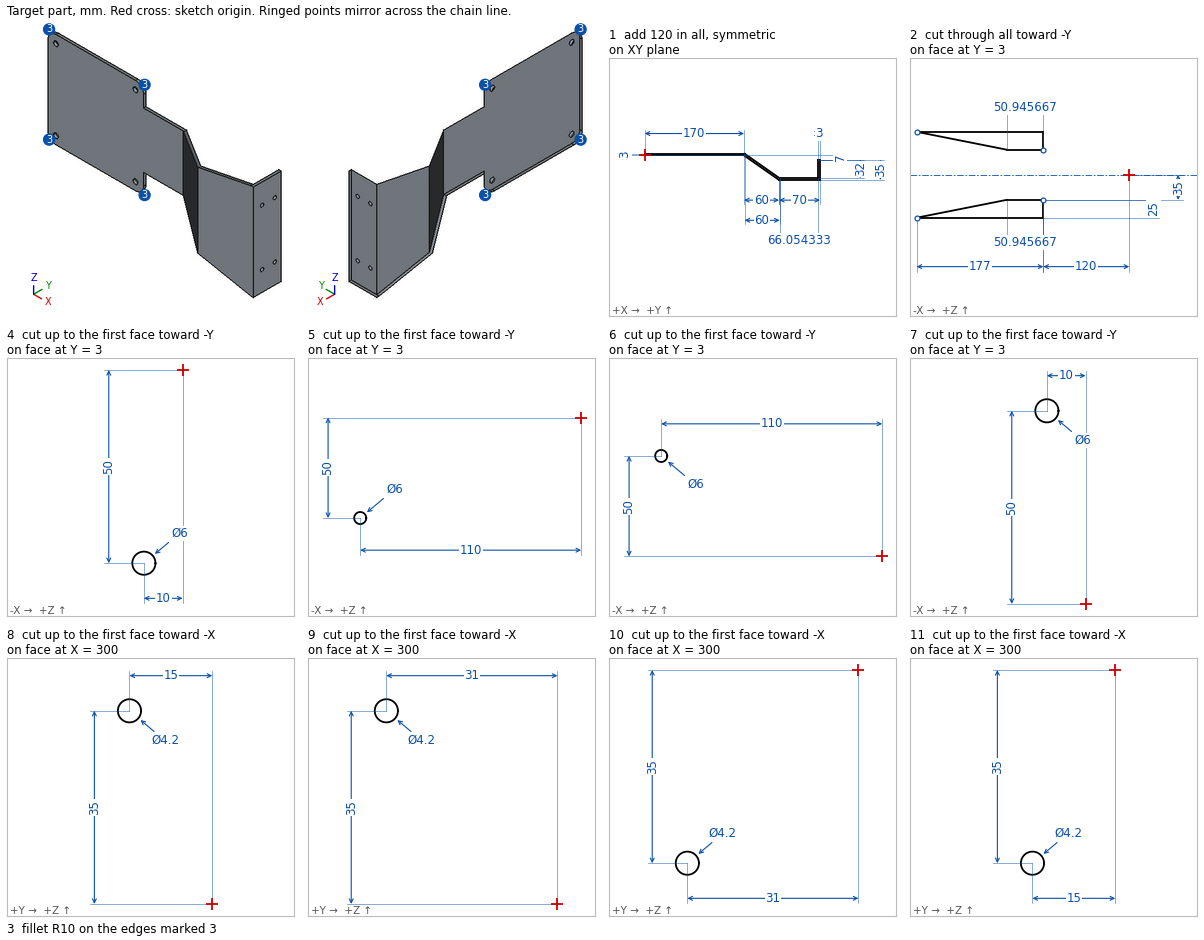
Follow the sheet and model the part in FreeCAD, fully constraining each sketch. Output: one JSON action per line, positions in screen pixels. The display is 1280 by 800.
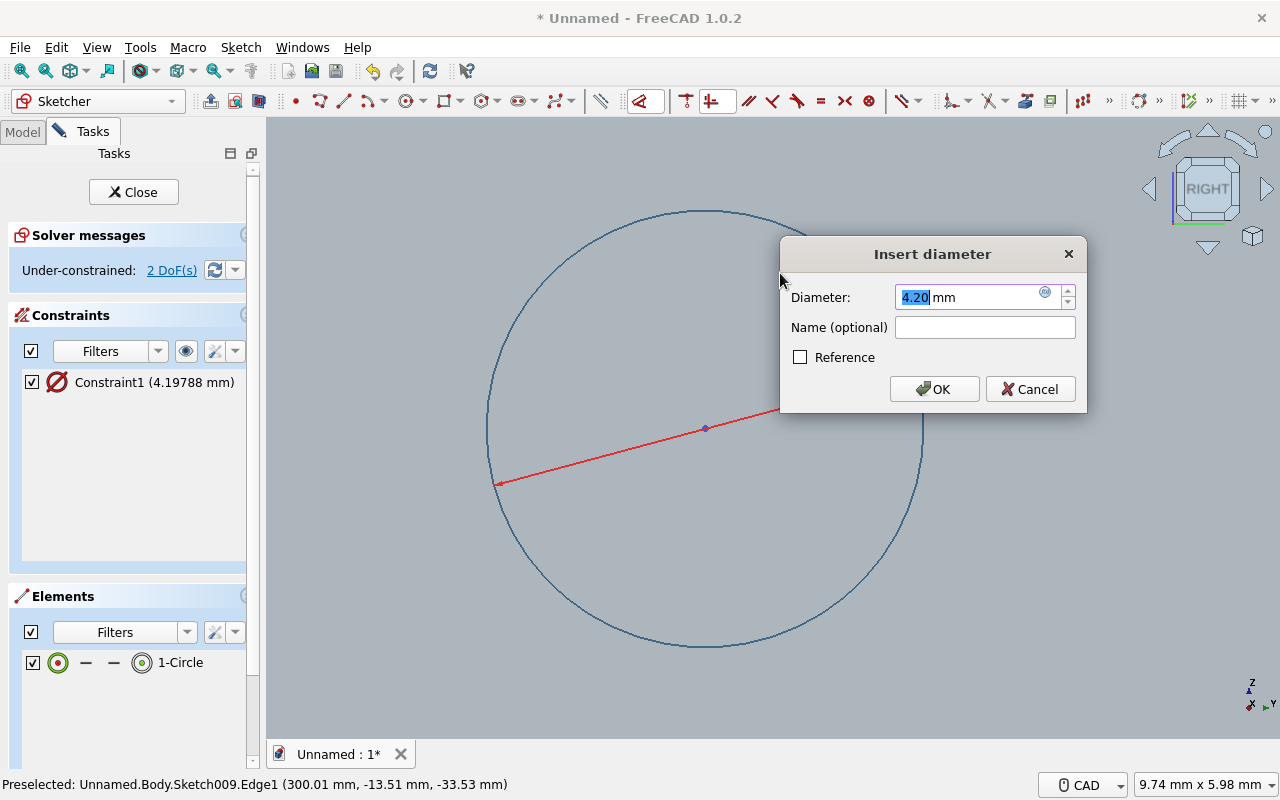
{"action": "type", "text": "4.2"}
{"action": "key", "text": "Return"}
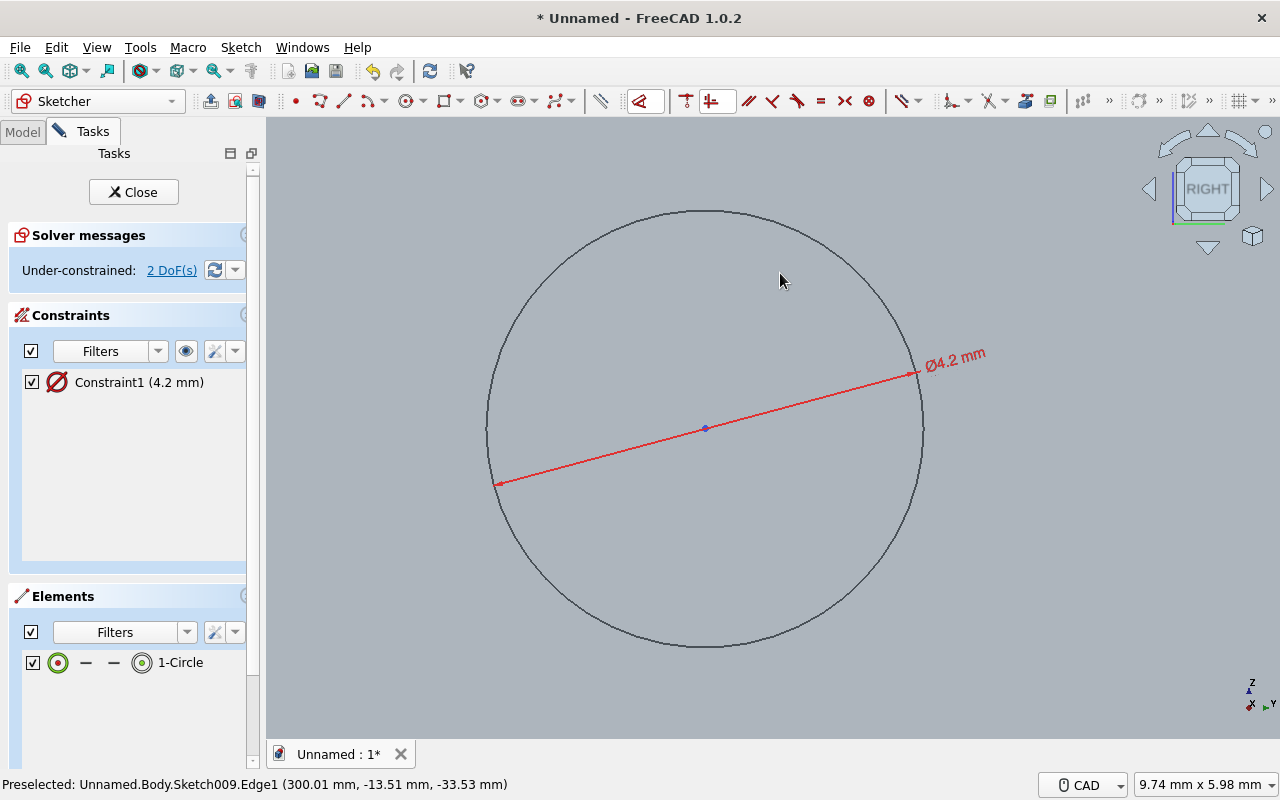
{"action": "left_click", "coordinate": [705, 429]}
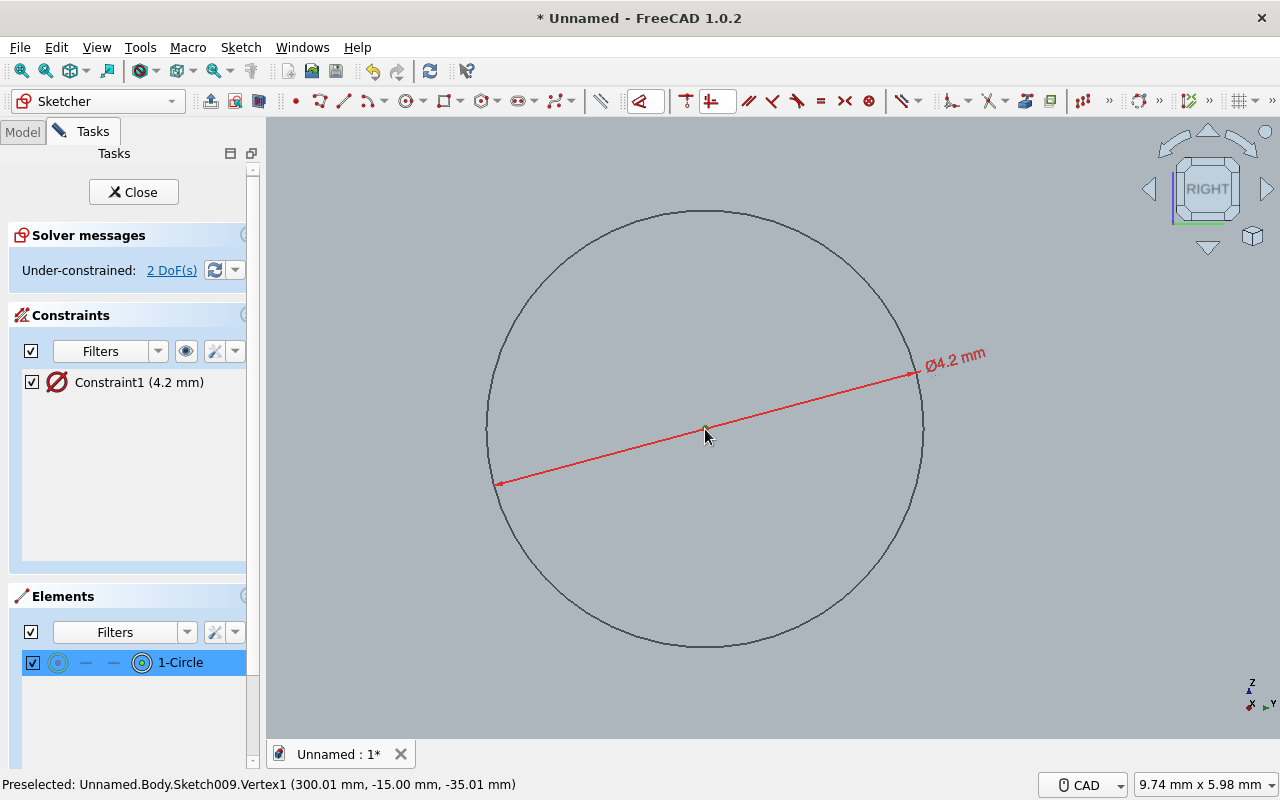
{"action": "key", "text": "l"}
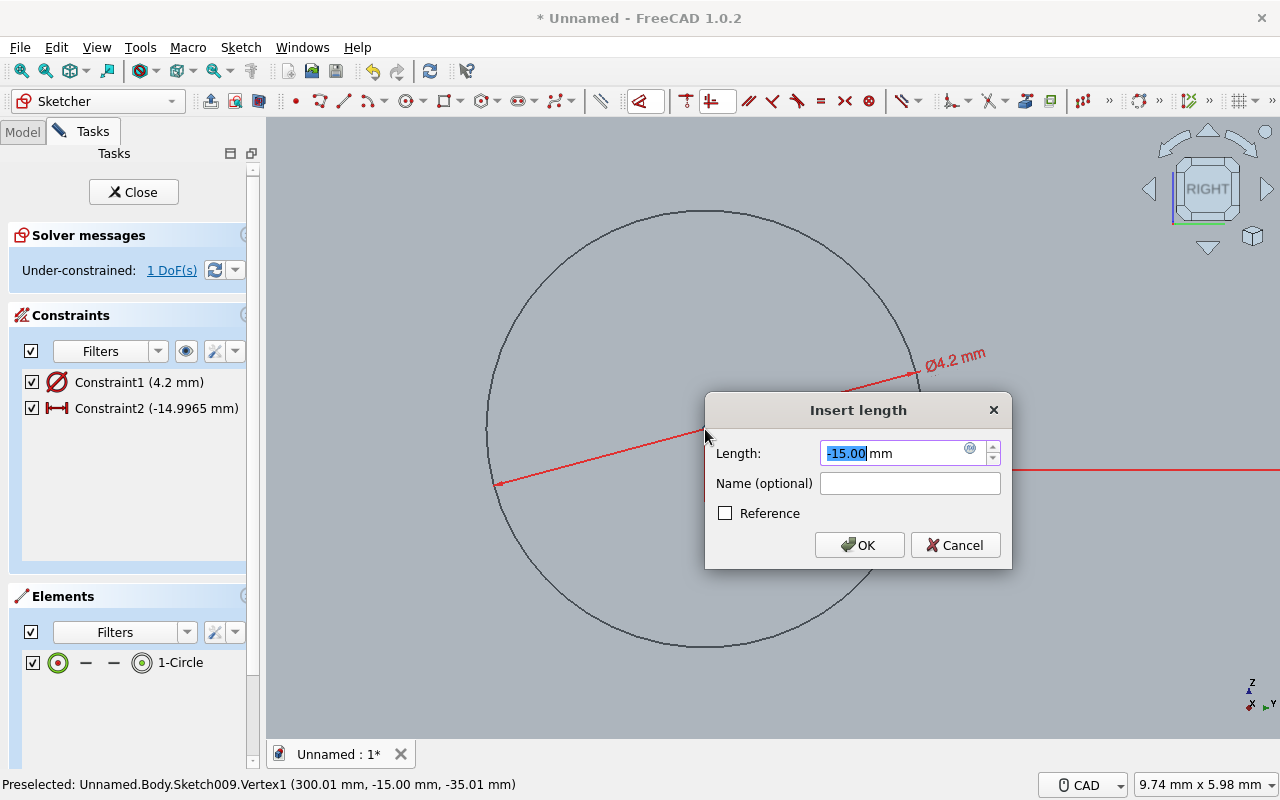
{"action": "type", "text": "-15"}
{"action": "key", "text": "Return"}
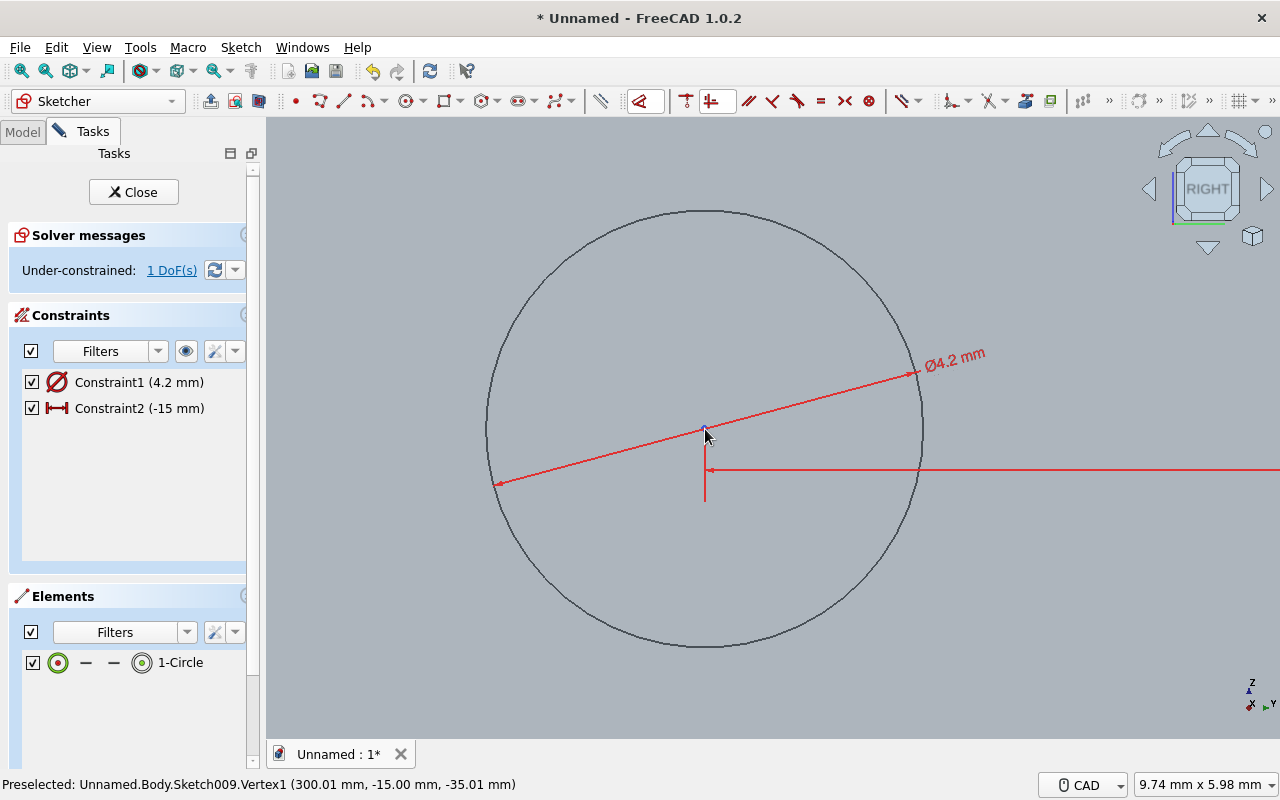
{"action": "left_click", "coordinate": [705, 429]}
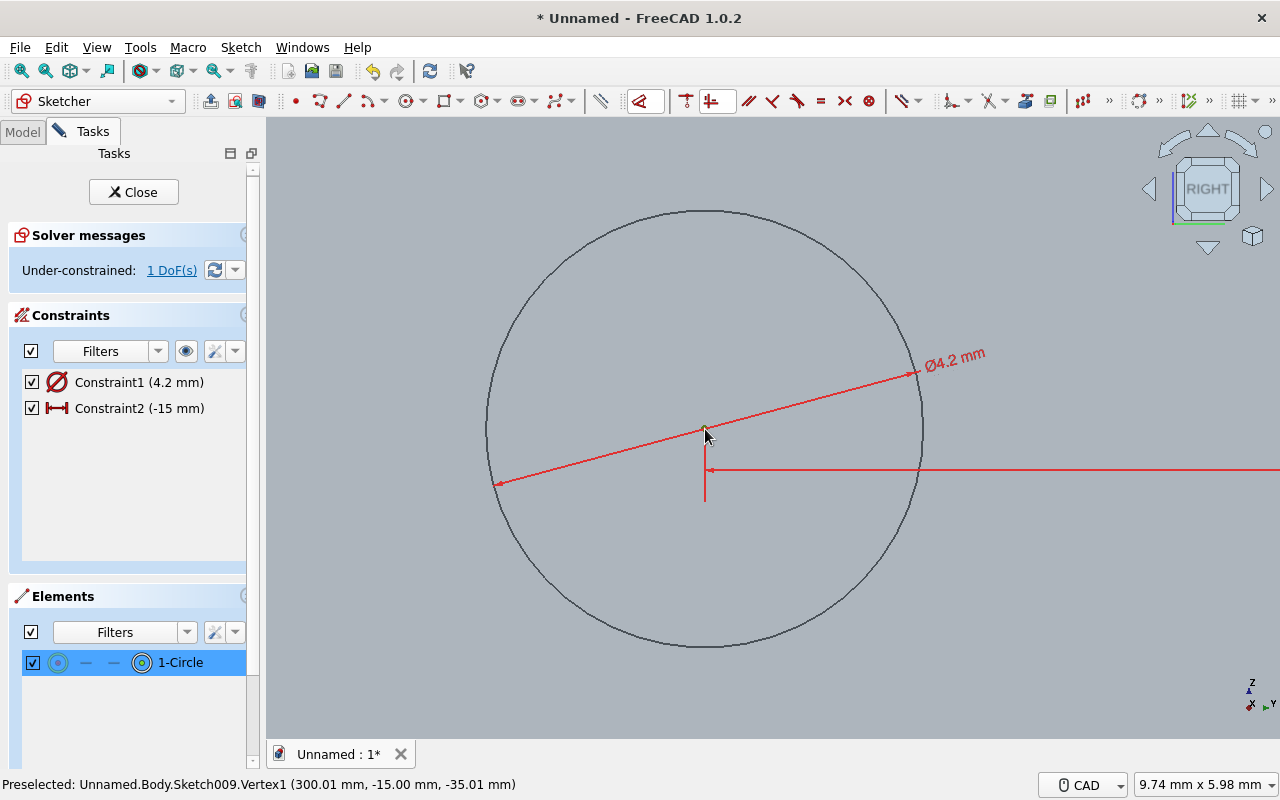
{"action": "left_click", "coordinate": [658, 102]}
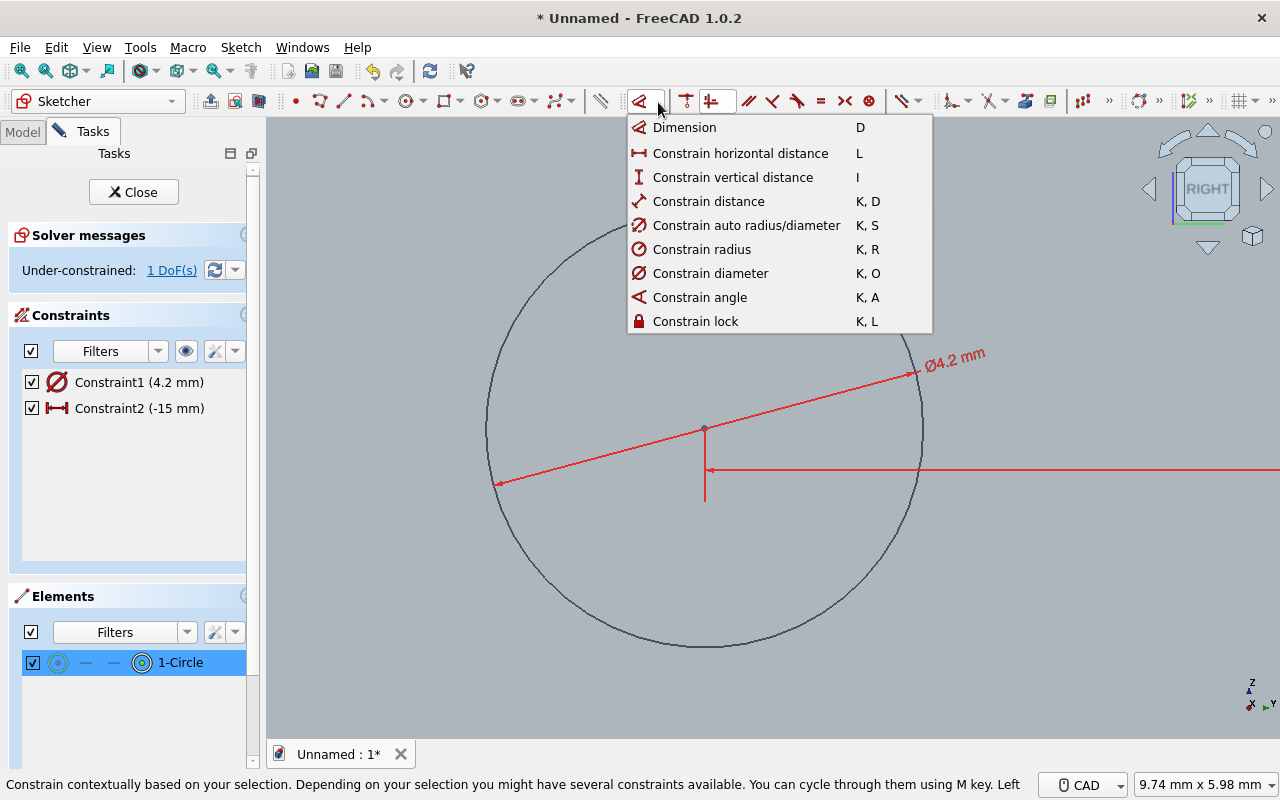
{"action": "left_click", "coordinate": [780, 177]}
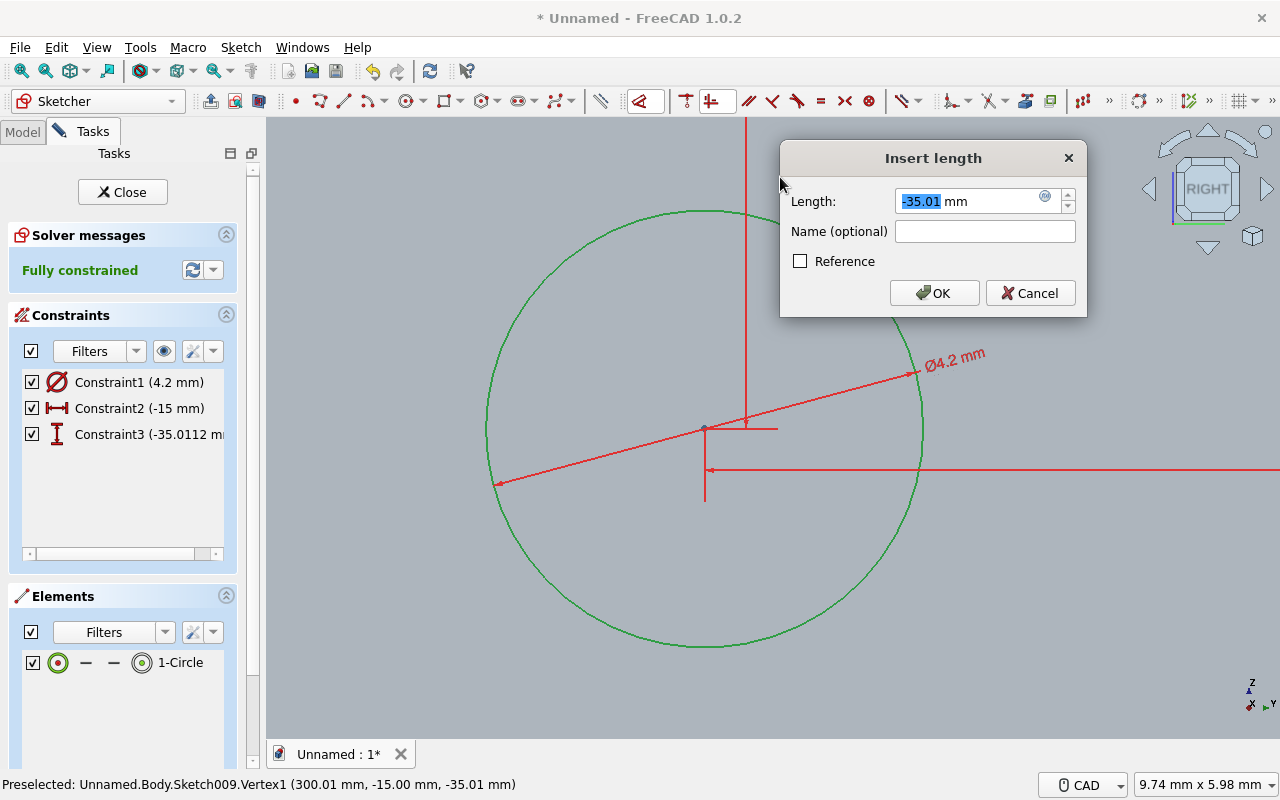
{"action": "type", "text": "-35"}
{"action": "key", "text": "Return"}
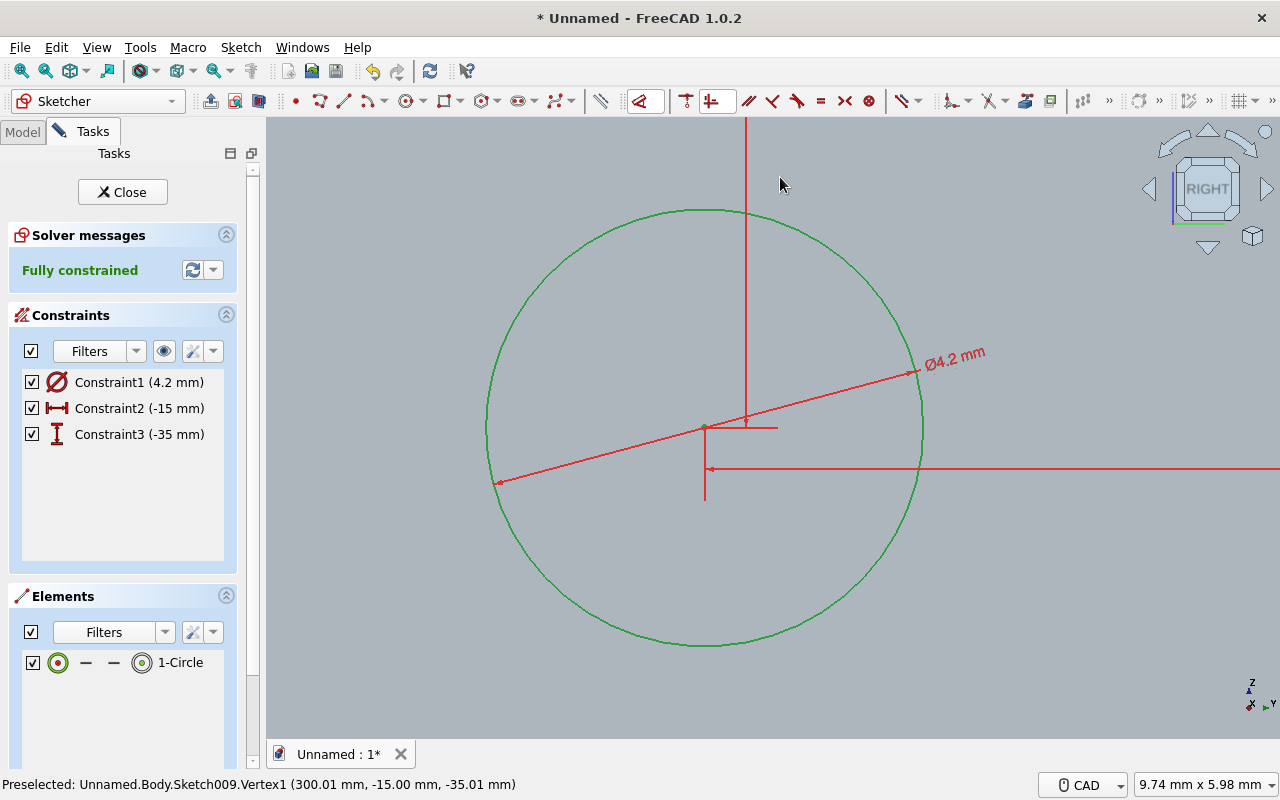
{"action": "left_click", "coordinate": [123, 192]}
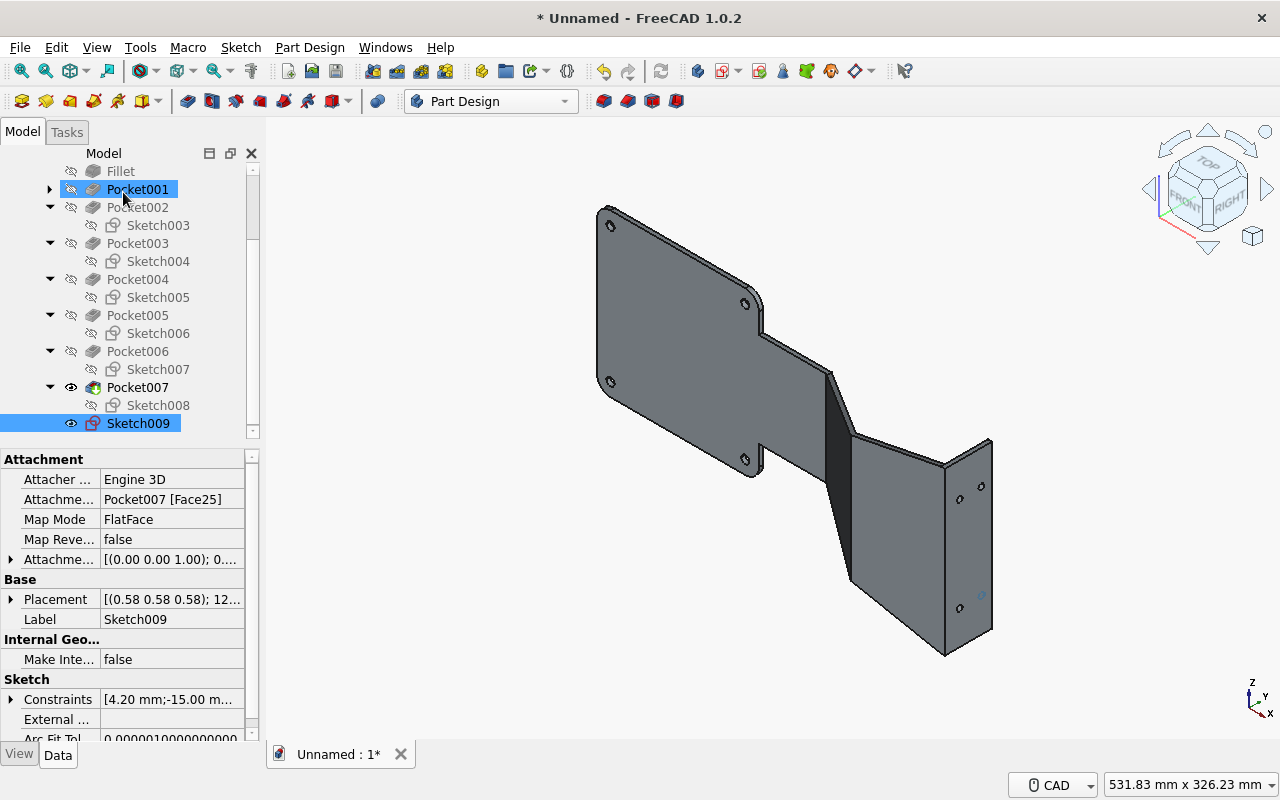
{"action": "left_click", "coordinate": [188, 102]}